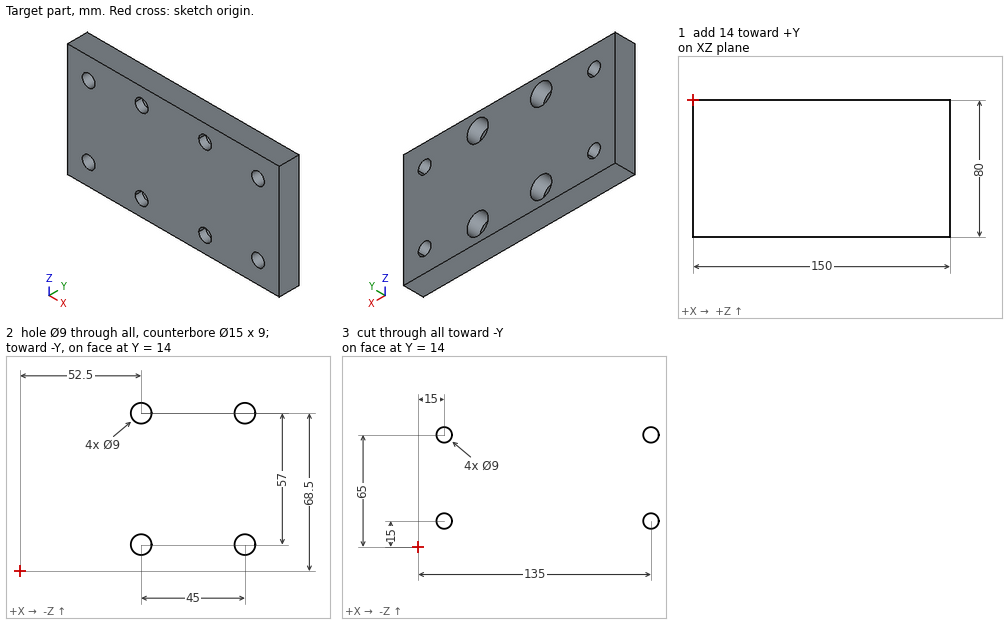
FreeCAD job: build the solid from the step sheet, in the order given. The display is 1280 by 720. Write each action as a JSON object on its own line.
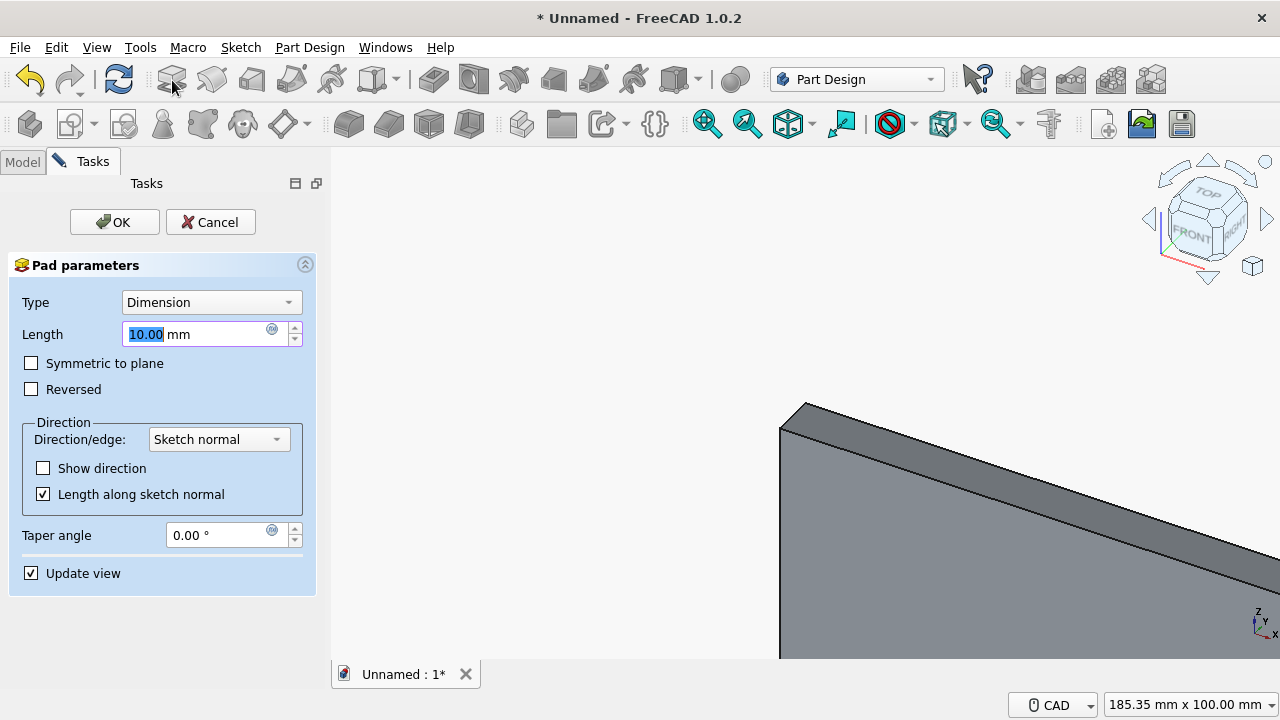
{"action": "type", "text": "14"}
{"action": "key", "text": "Tab"}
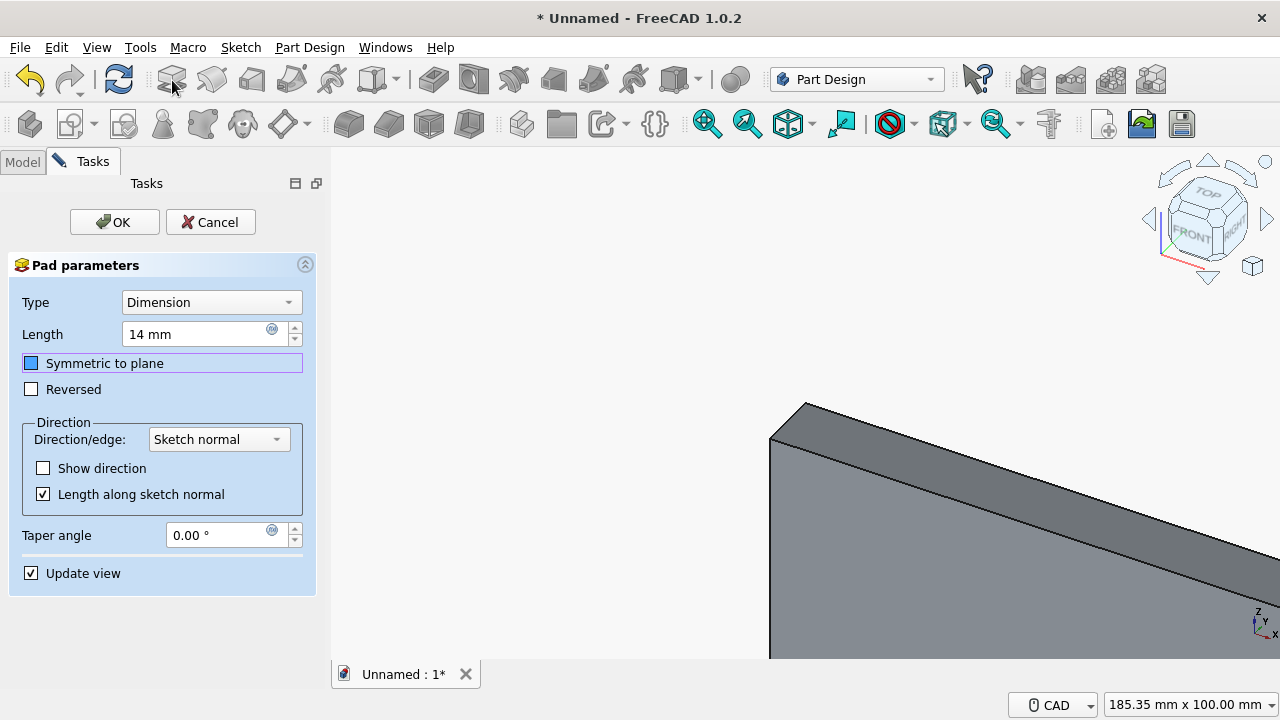
{"action": "left_click", "coordinate": [30, 389]}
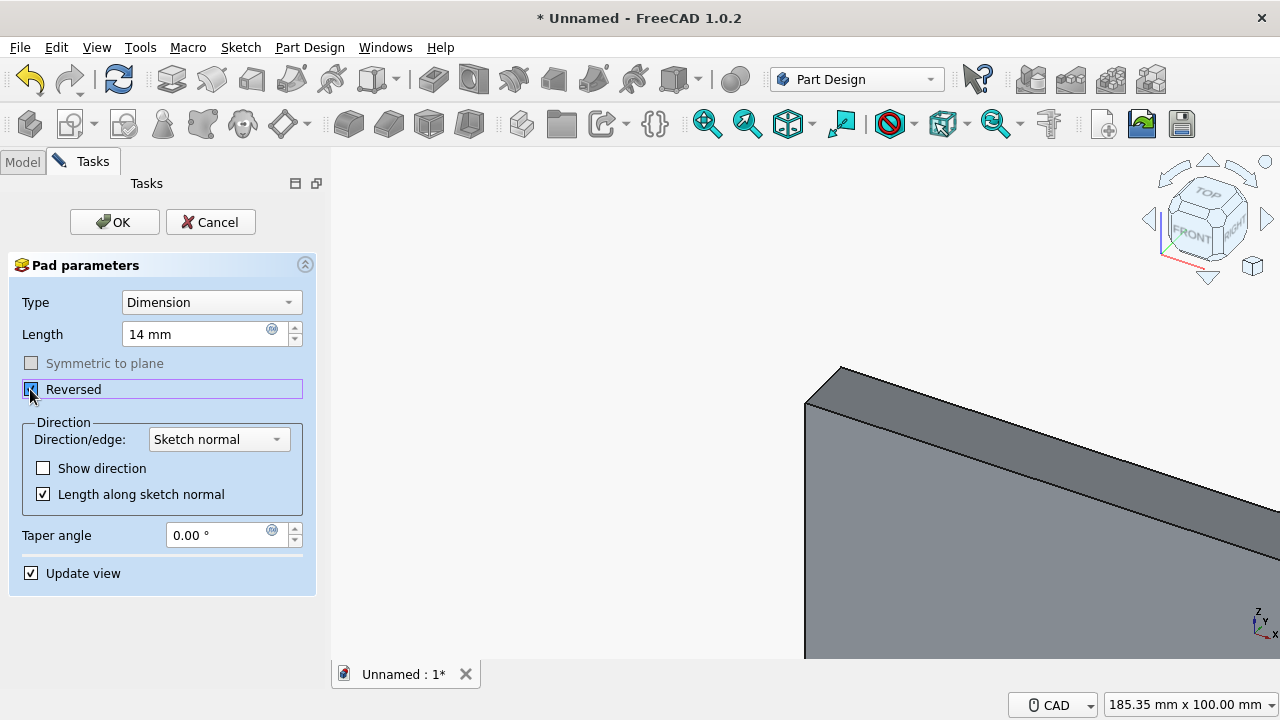
{"action": "left_click", "coordinate": [115, 222]}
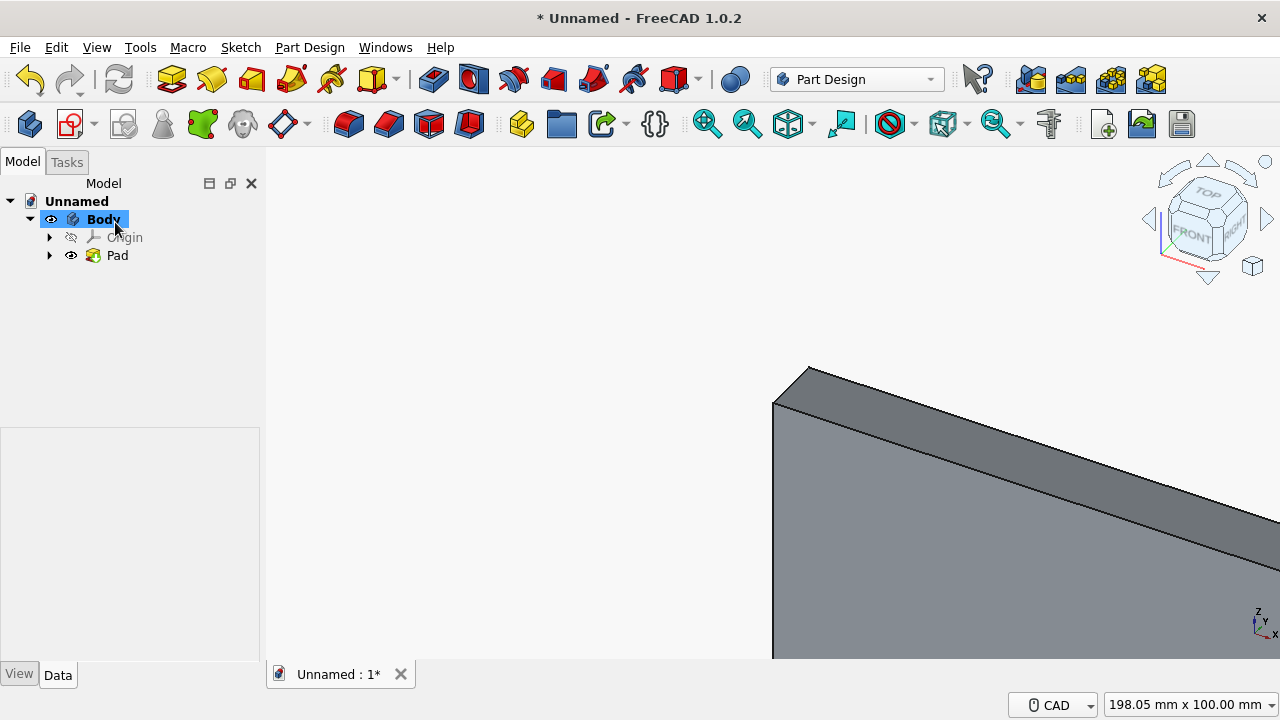
{"action": "left_click", "coordinate": [708, 124]}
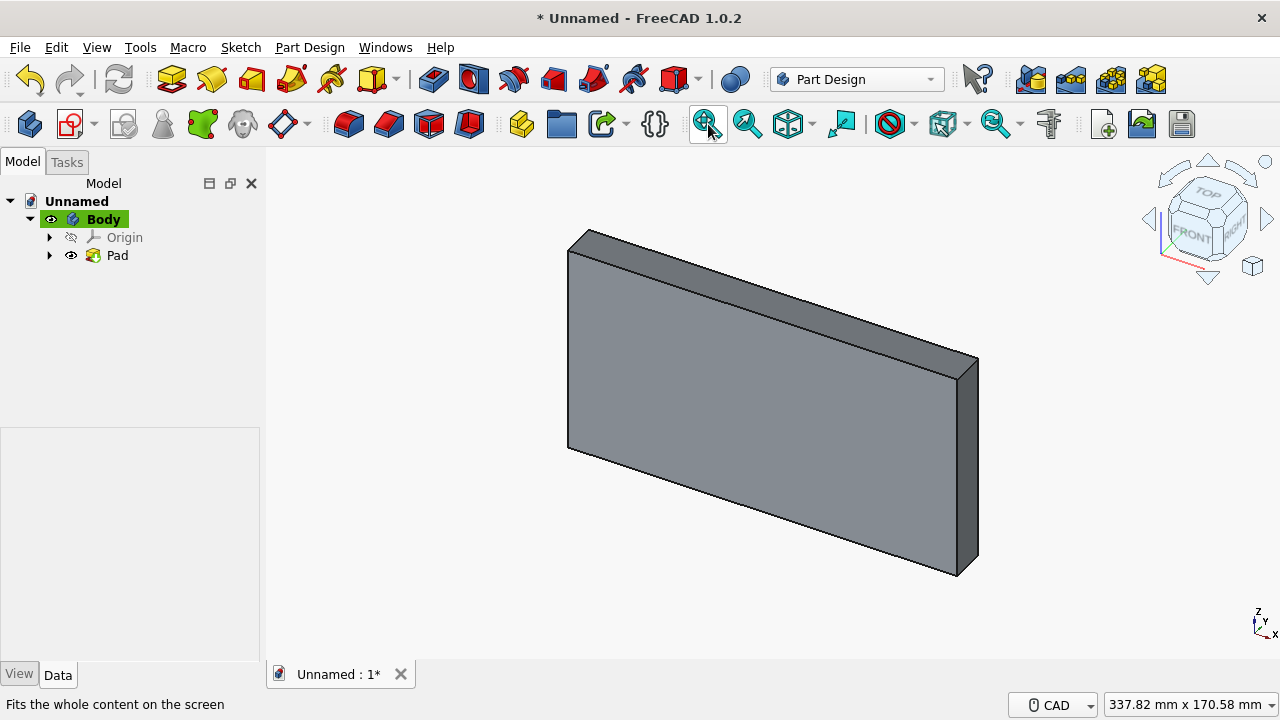
{"action": "key", "text": "4"}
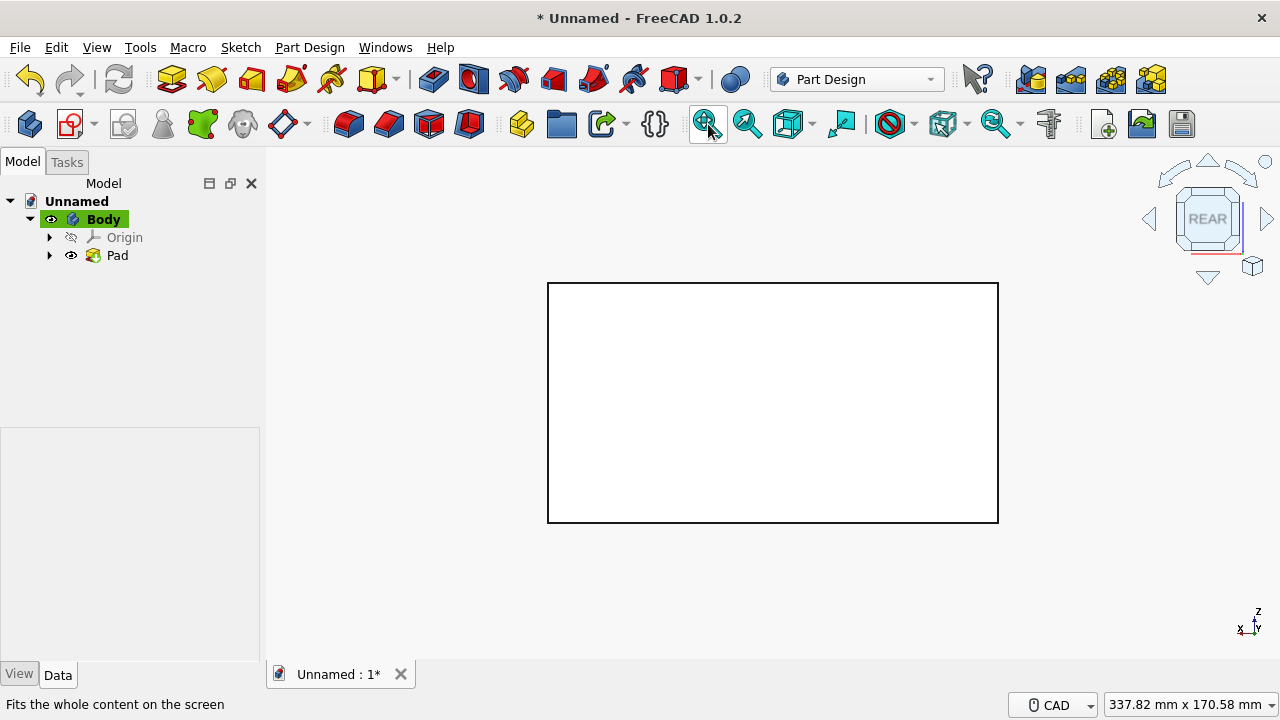
{"action": "left_click", "coordinate": [709, 402]}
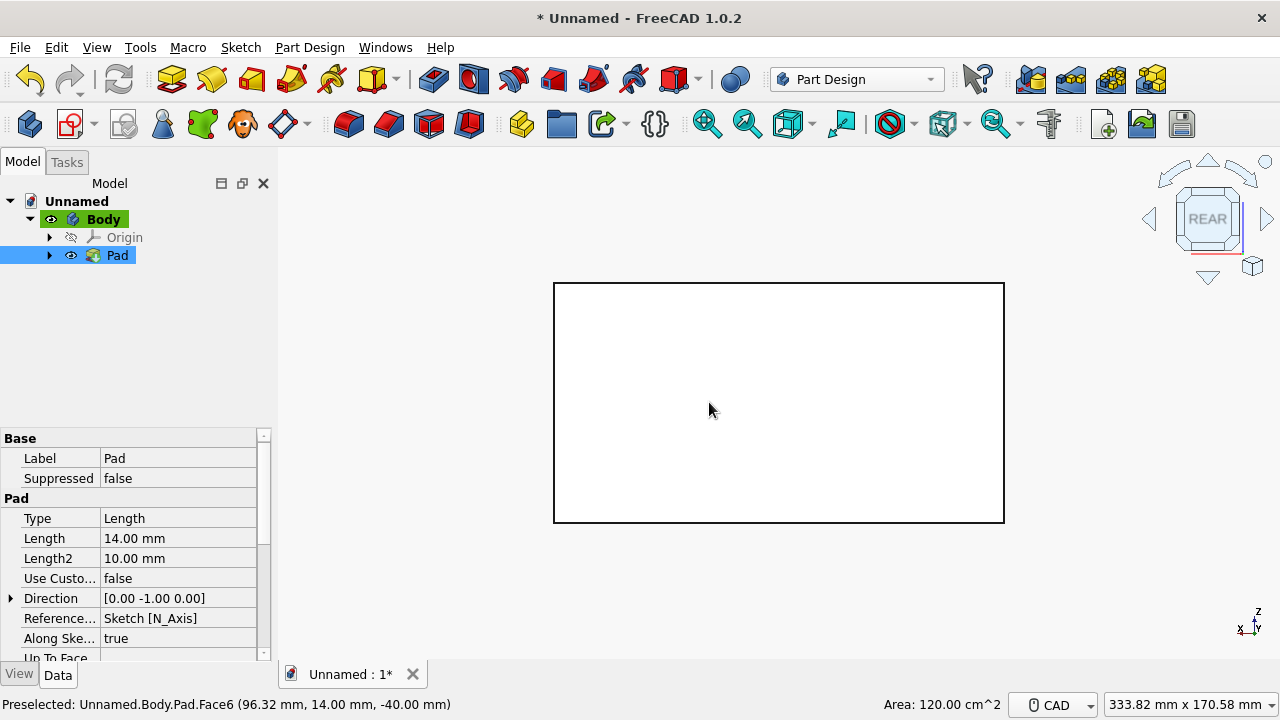
{"action": "left_click", "coordinate": [70, 124]}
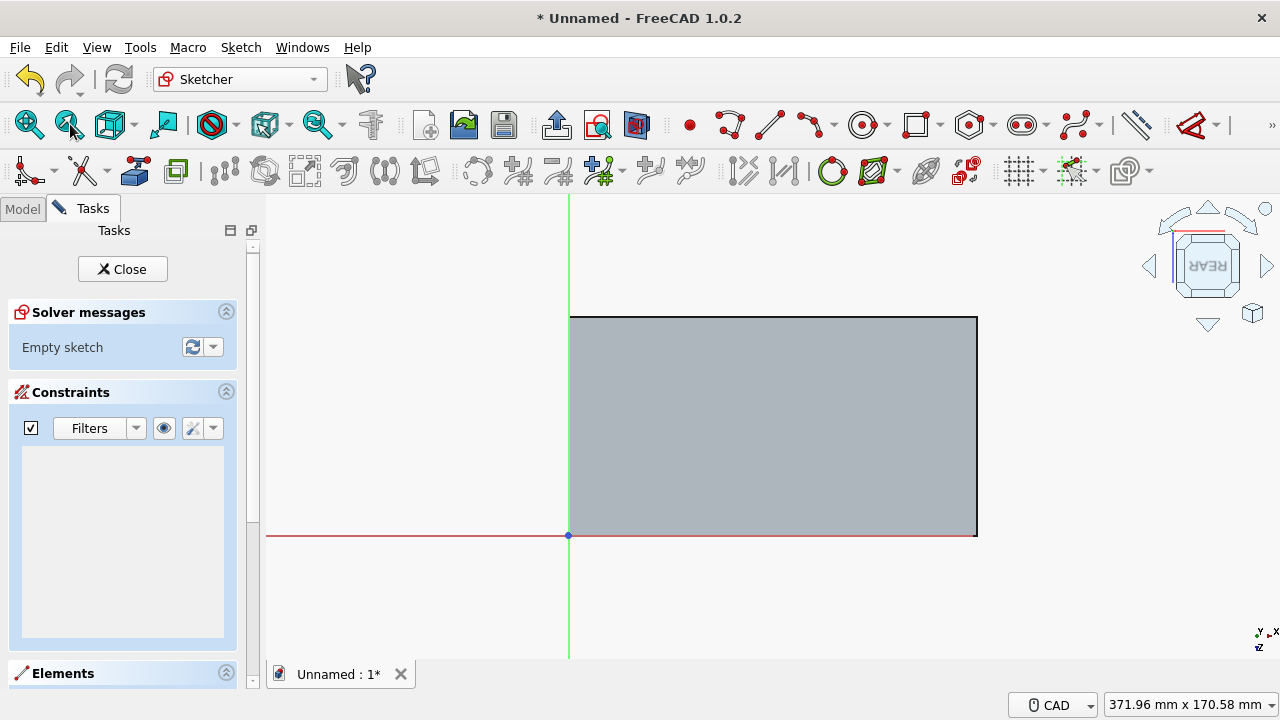
{"action": "scroll", "coordinate": [714, 455], "scroll_direction": "up", "scroll_amount": 2}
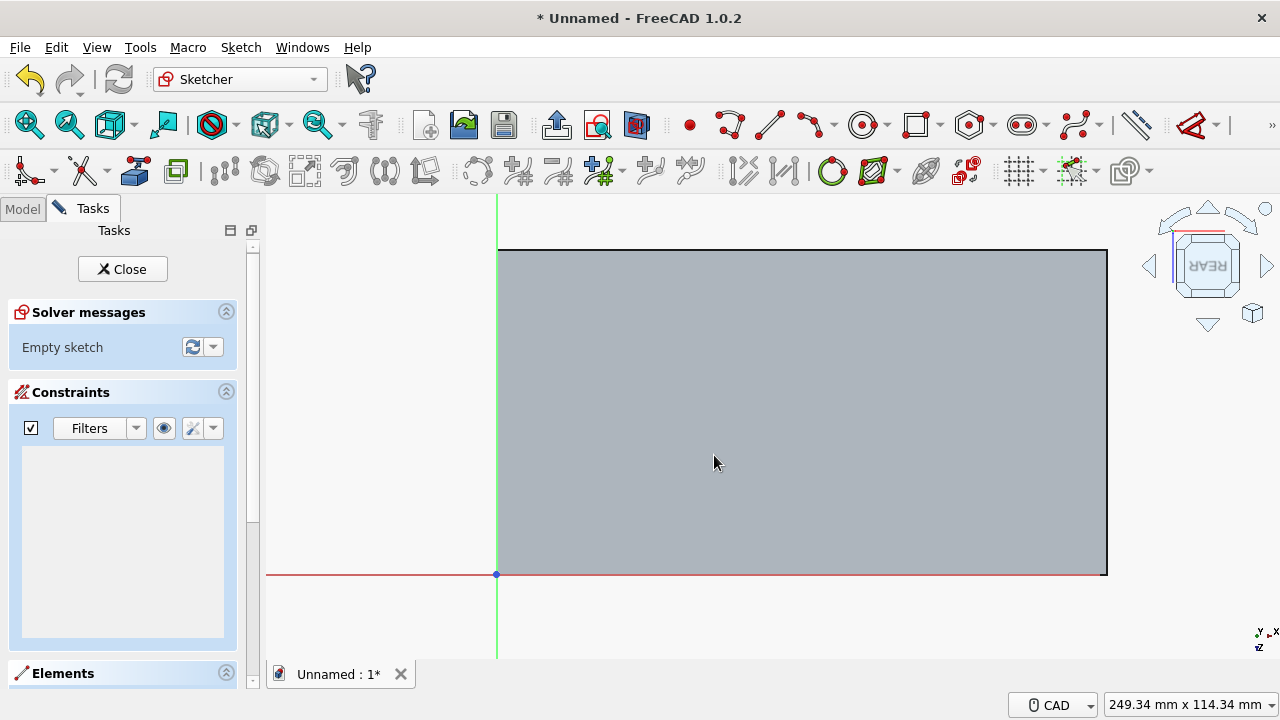
{"action": "left_click", "coordinate": [864, 126]}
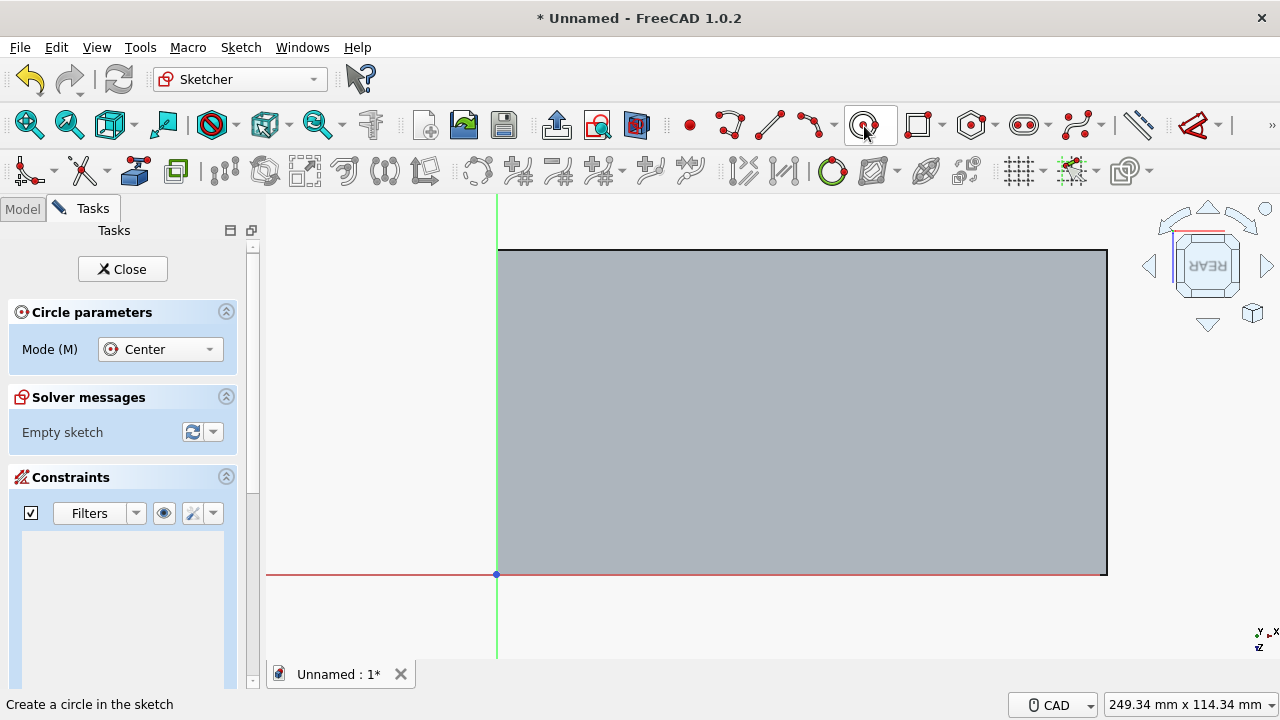
{"action": "scroll", "coordinate": [710, 296], "scroll_direction": "up", "scroll_amount": 2}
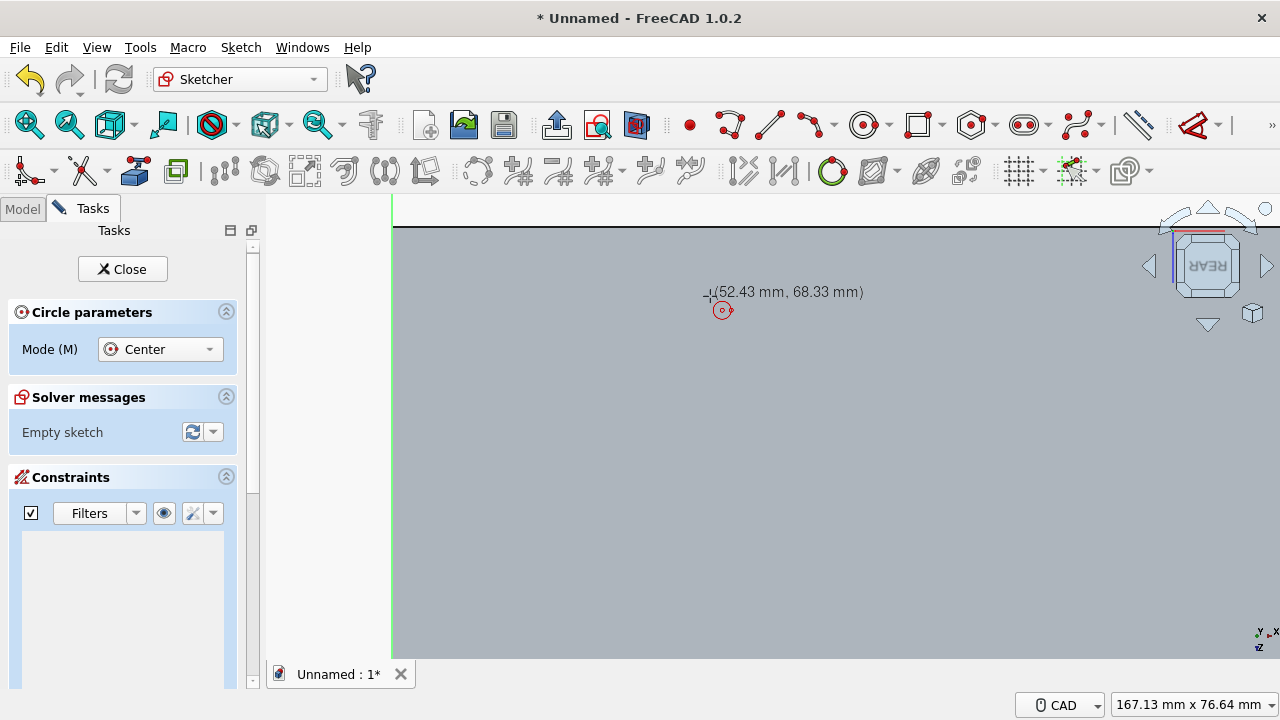
{"action": "left_click", "coordinate": [710, 296]}
{"action": "mouse_move", "coordinate": [730, 277]}